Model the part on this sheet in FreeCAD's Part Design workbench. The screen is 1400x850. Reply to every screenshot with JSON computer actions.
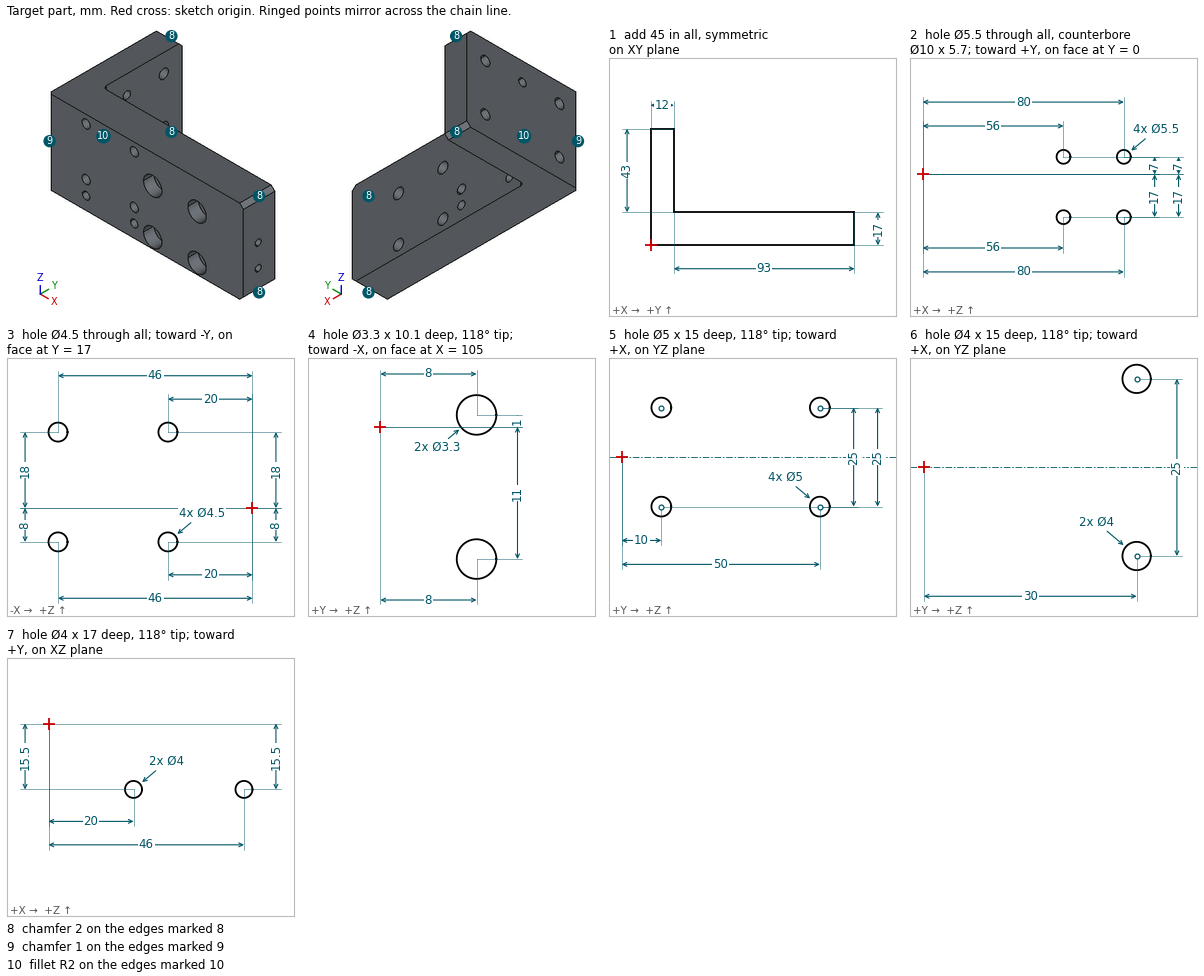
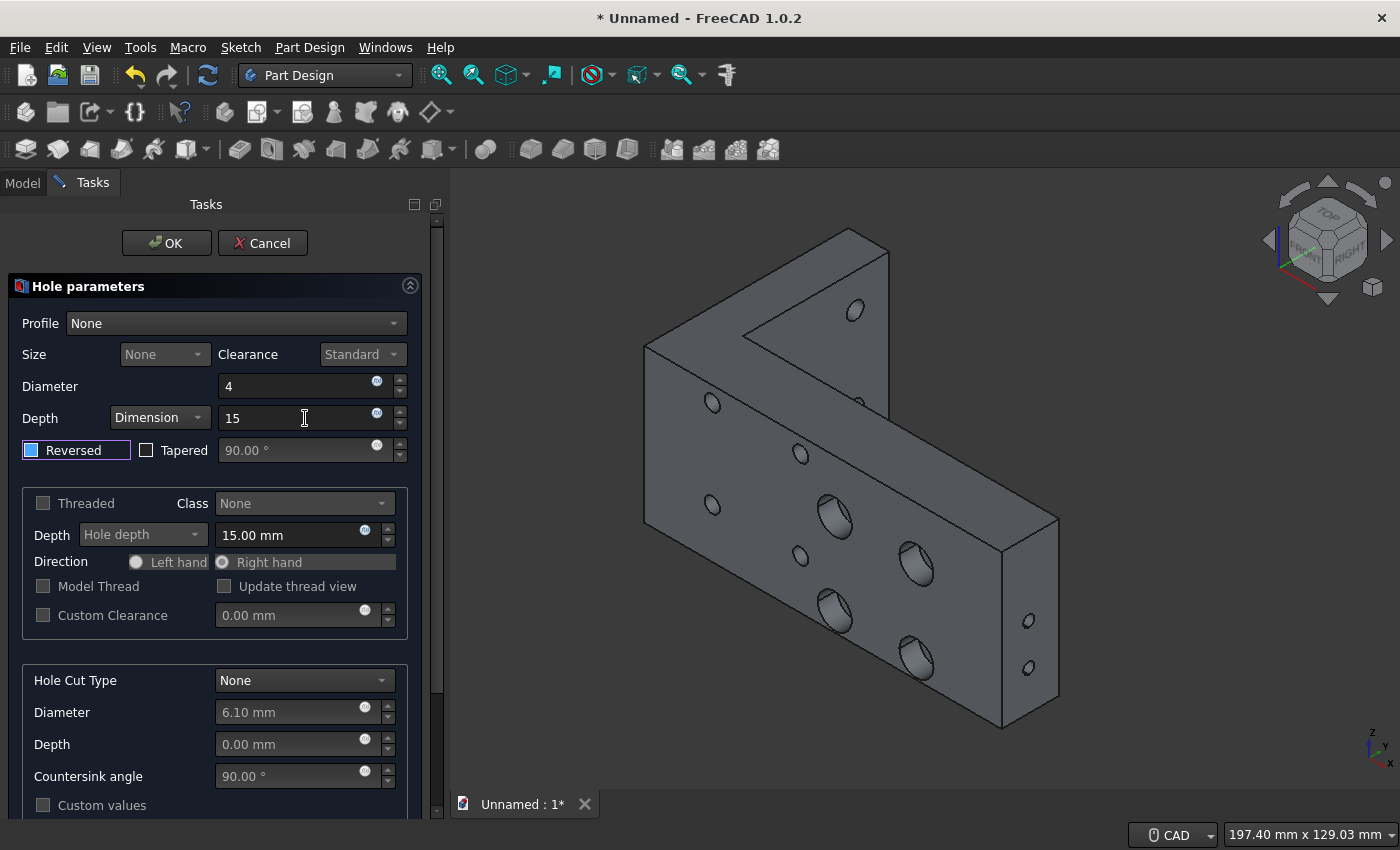
{"action": "left_click", "coordinate": [30, 450]}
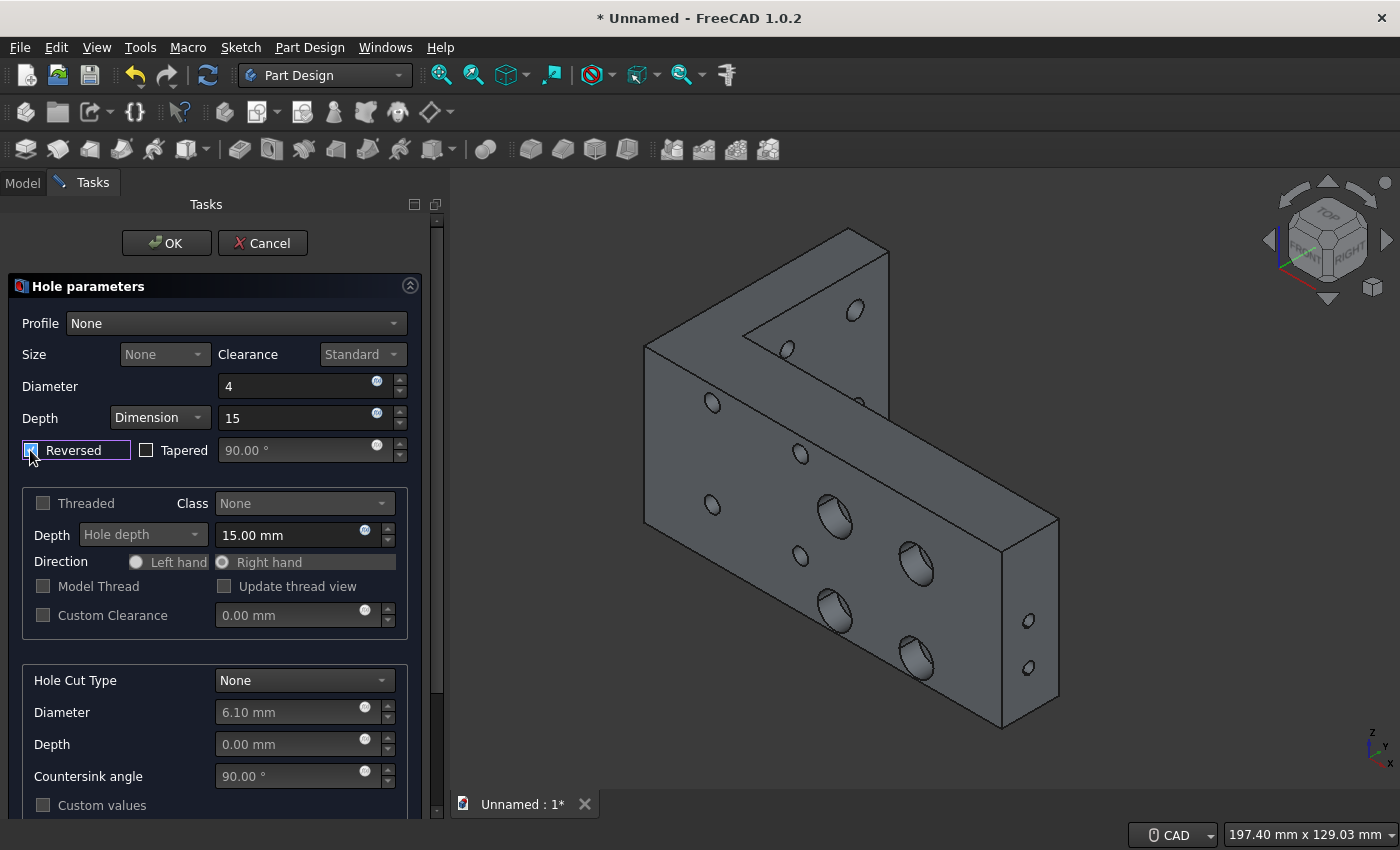
{"action": "left_click", "coordinate": [167, 243]}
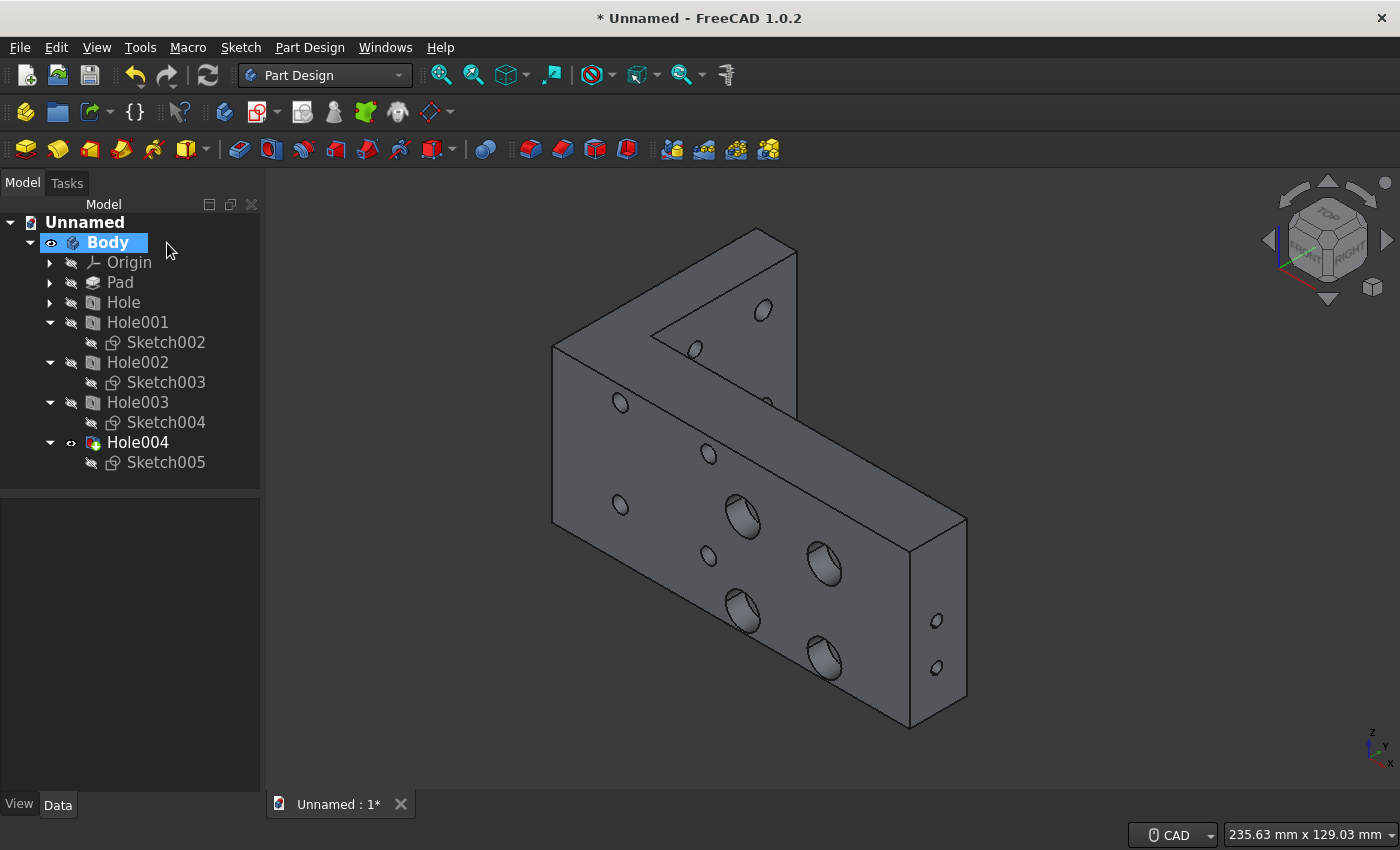
{"action": "left_click", "coordinate": [258, 112]}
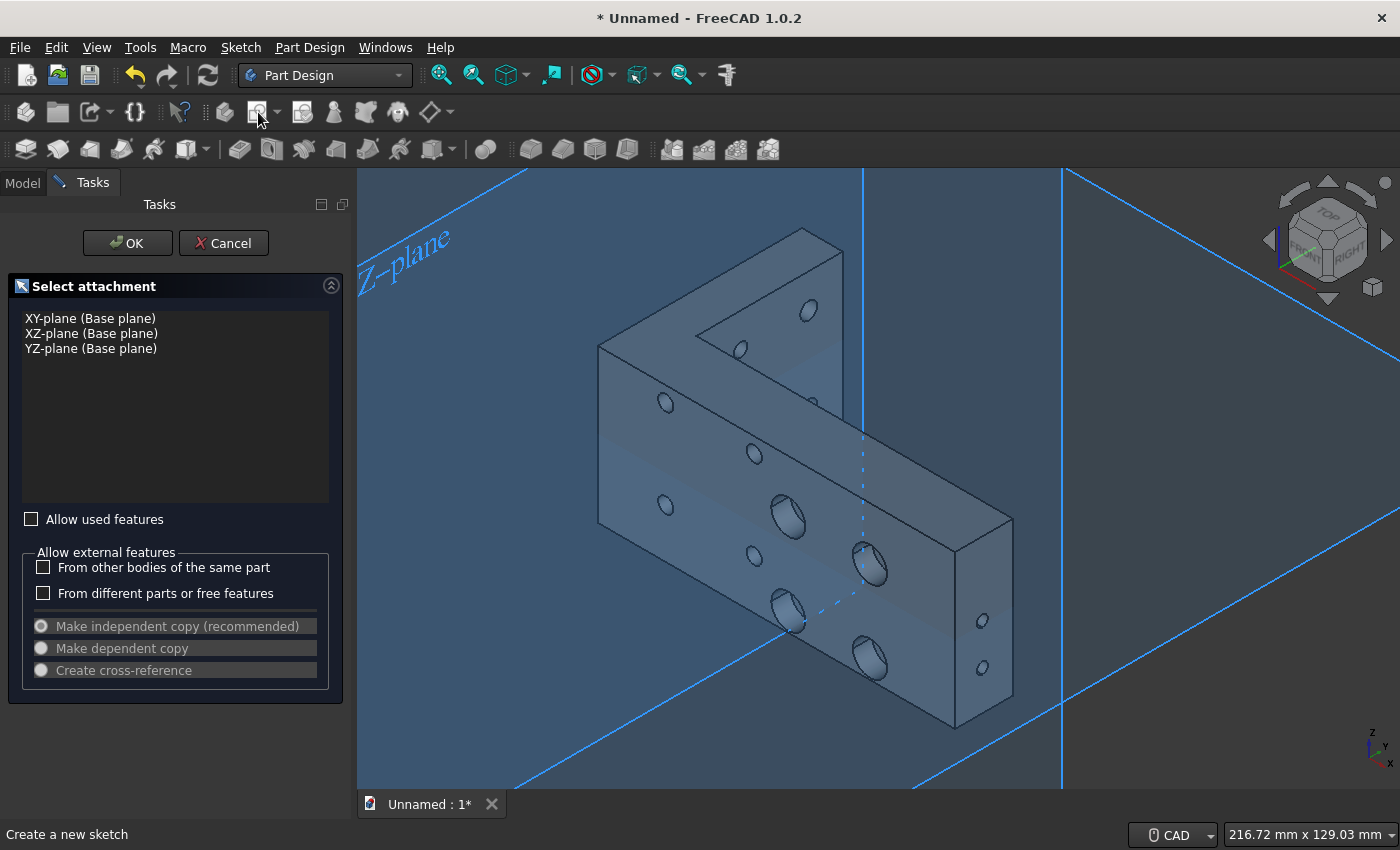
{"action": "left_click", "coordinate": [82, 334]}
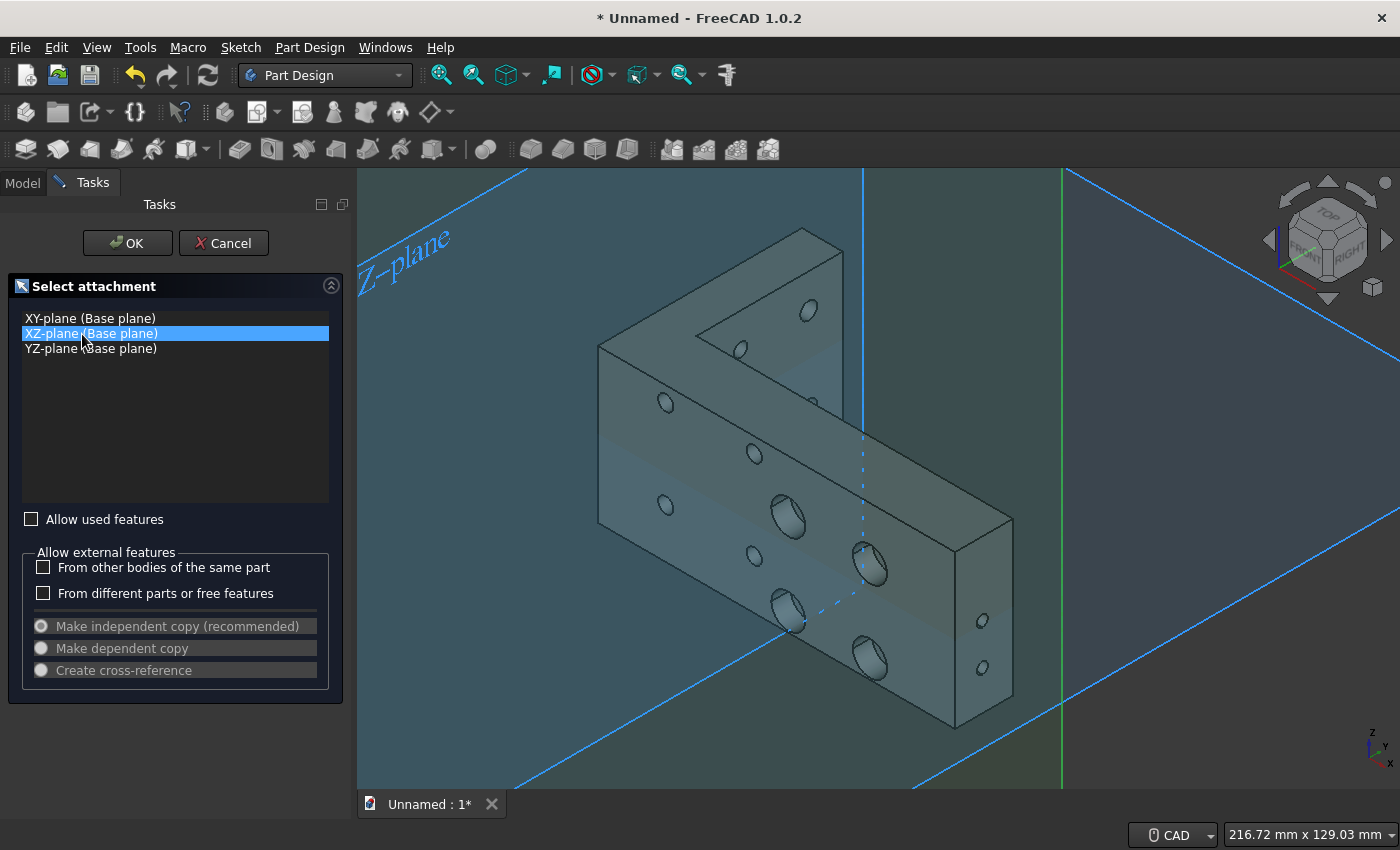
{"action": "left_click", "coordinate": [128, 243]}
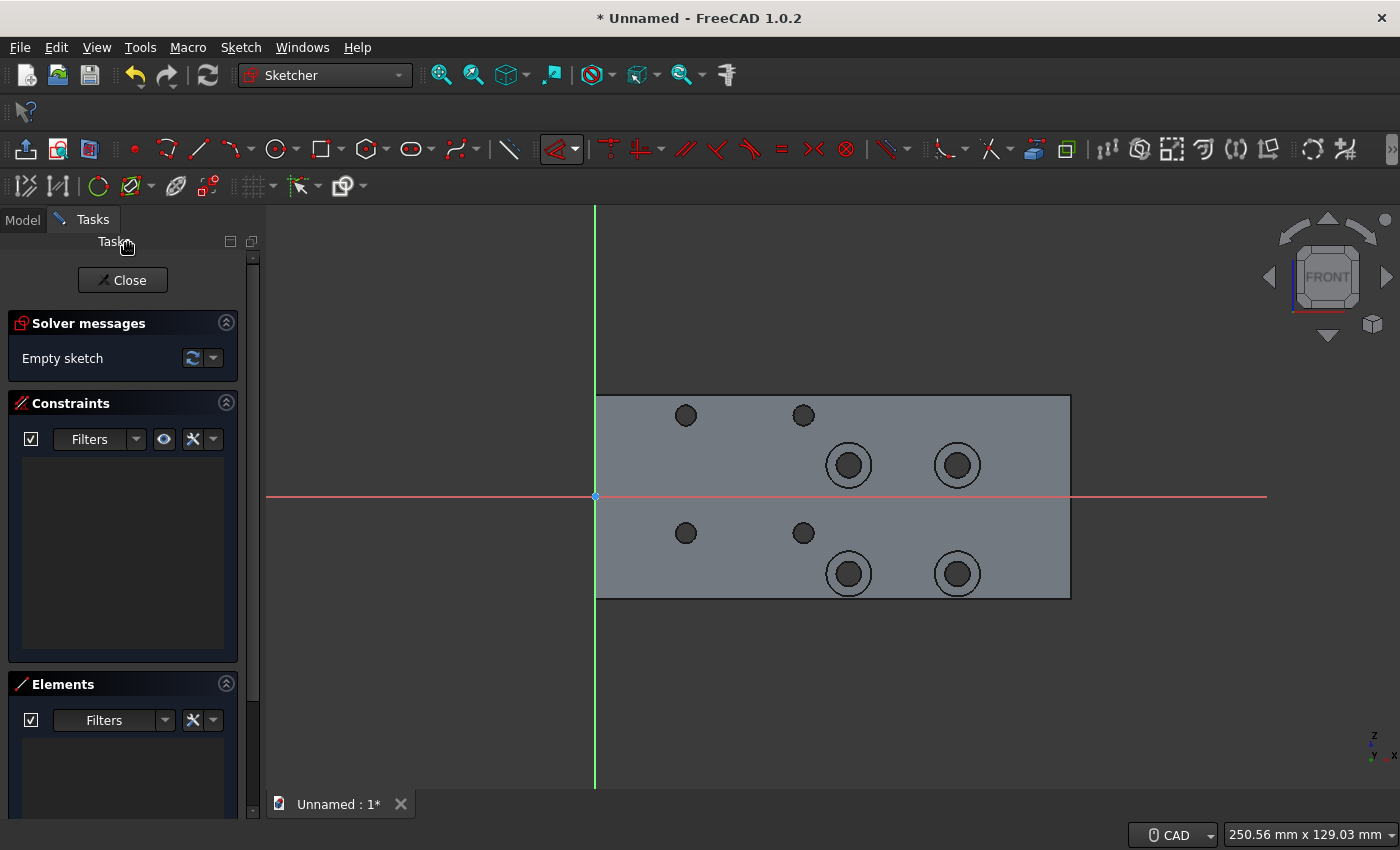
{"action": "scroll", "coordinate": [678, 554], "scroll_direction": "up", "scroll_amount": 6}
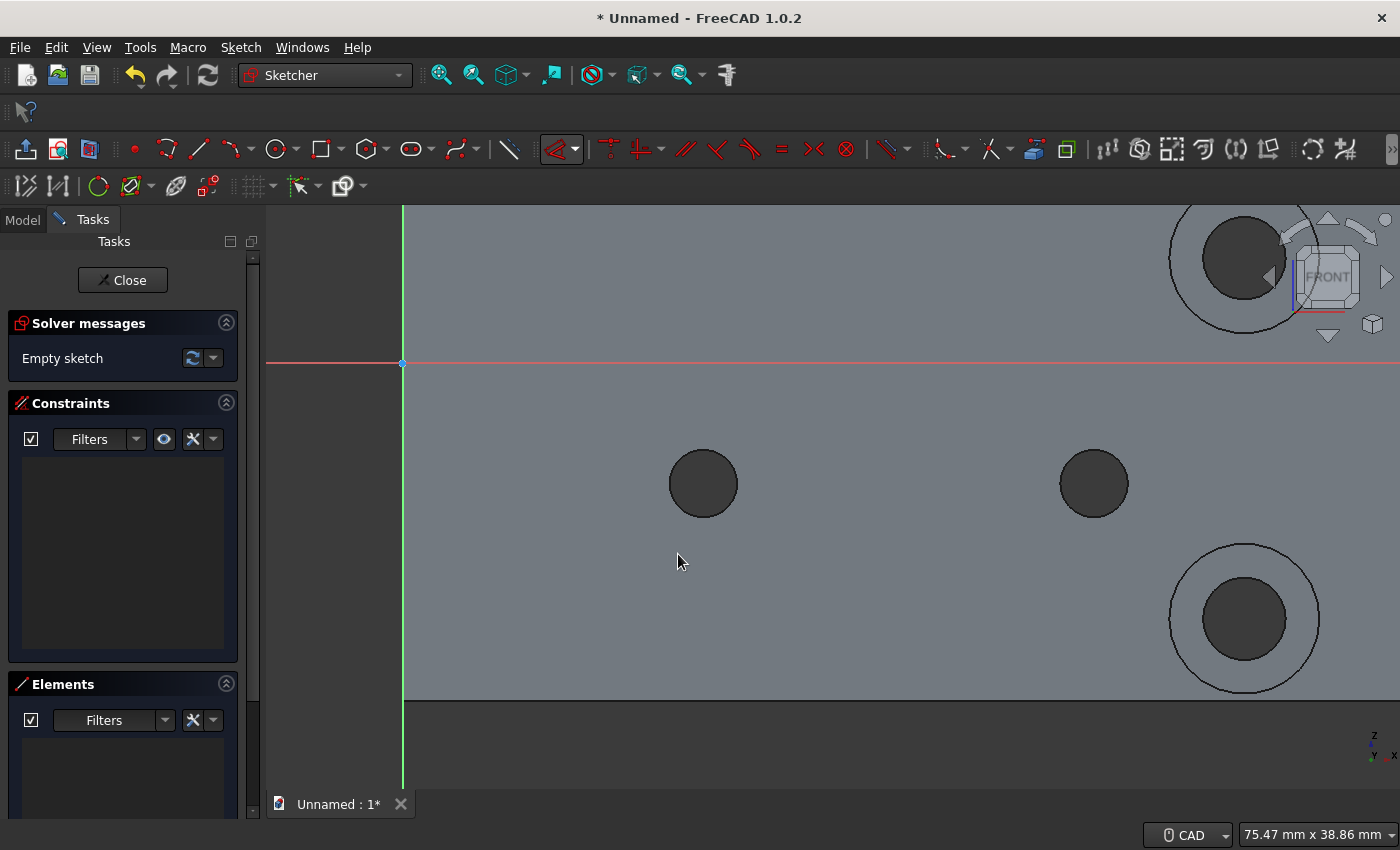
{"action": "key", "text": "g c"}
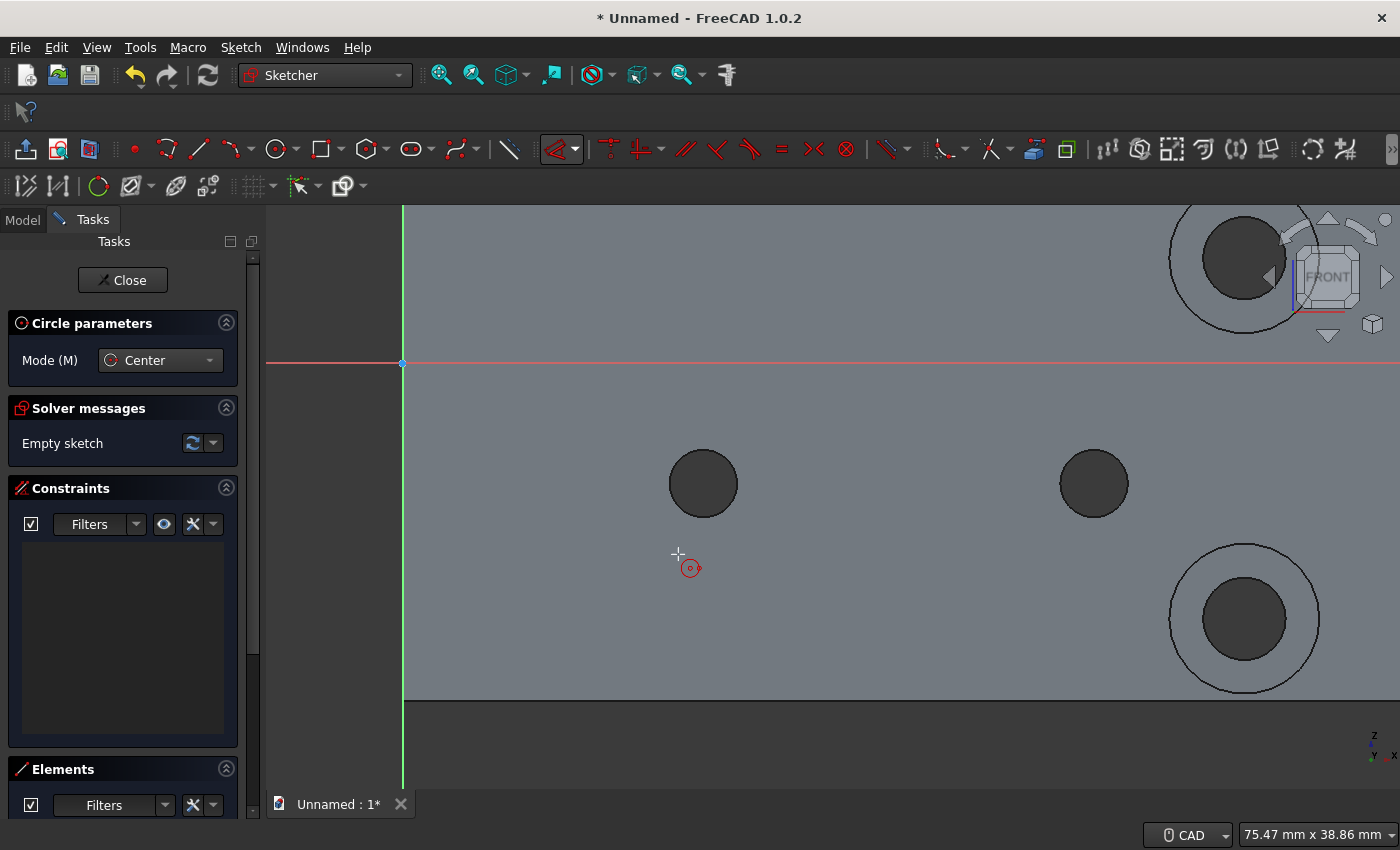
{"action": "left_click", "coordinate": [703, 596]}
{"action": "left_click", "coordinate": [725, 575]}